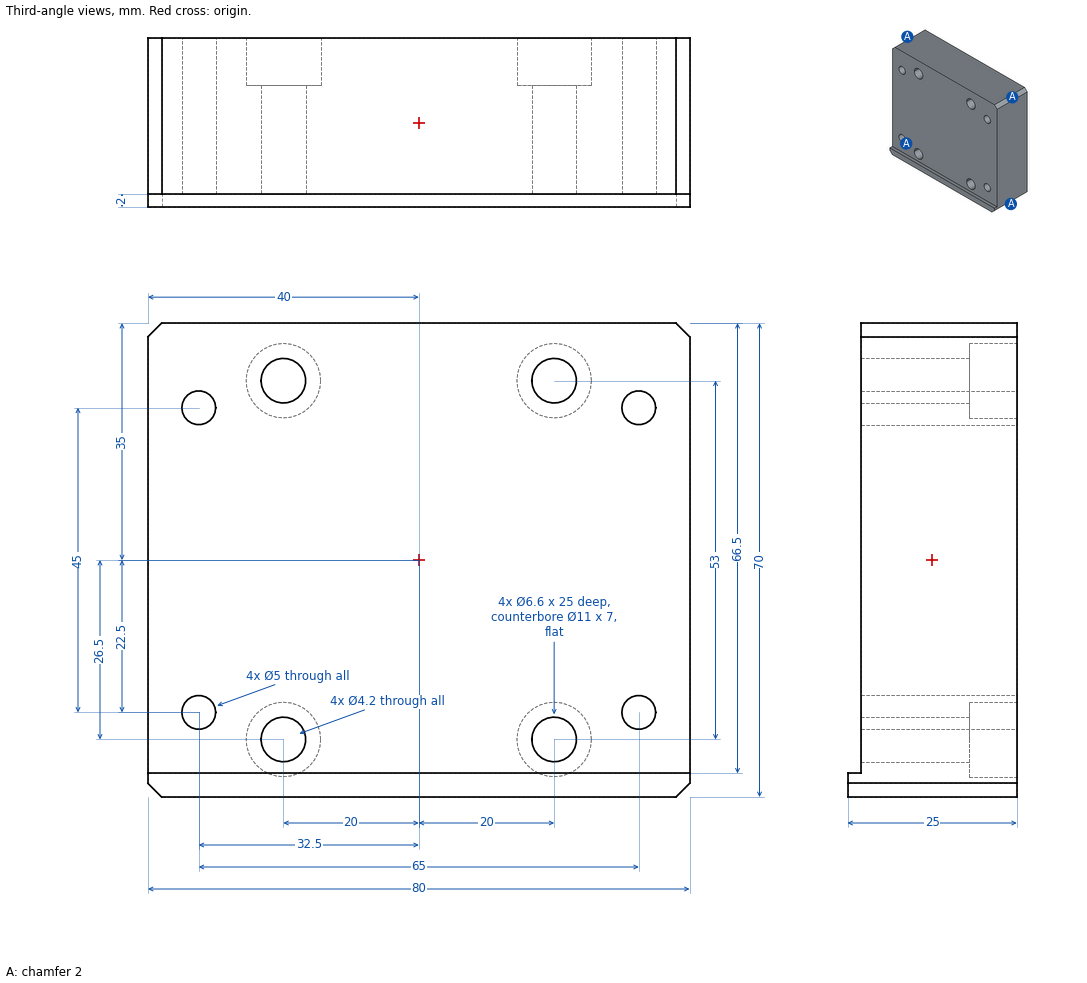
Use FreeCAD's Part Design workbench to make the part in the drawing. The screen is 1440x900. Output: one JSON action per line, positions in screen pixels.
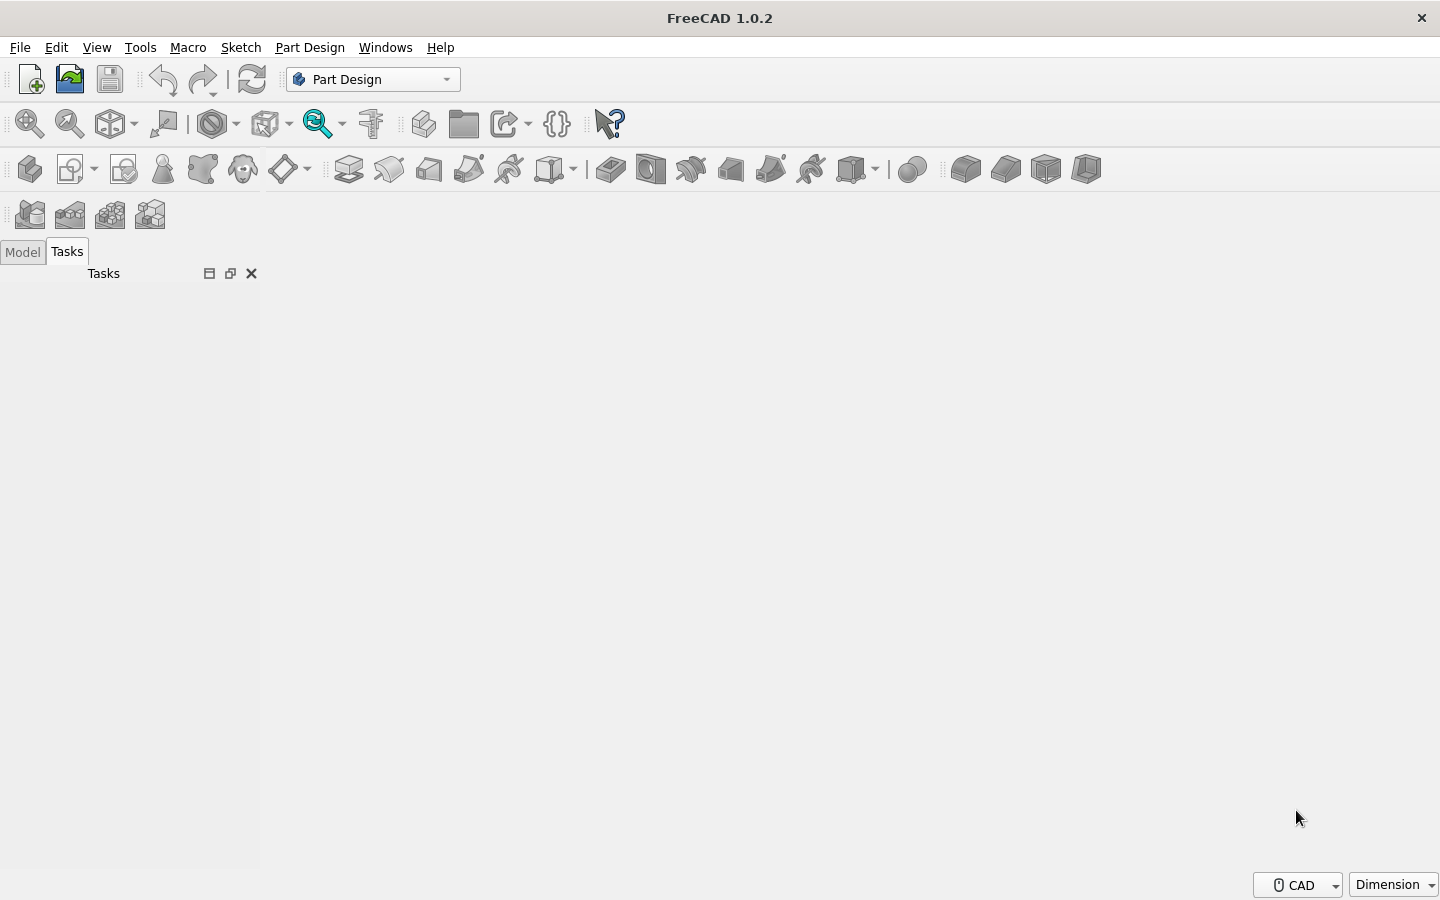
{"action": "left_click", "coordinate": [30, 80]}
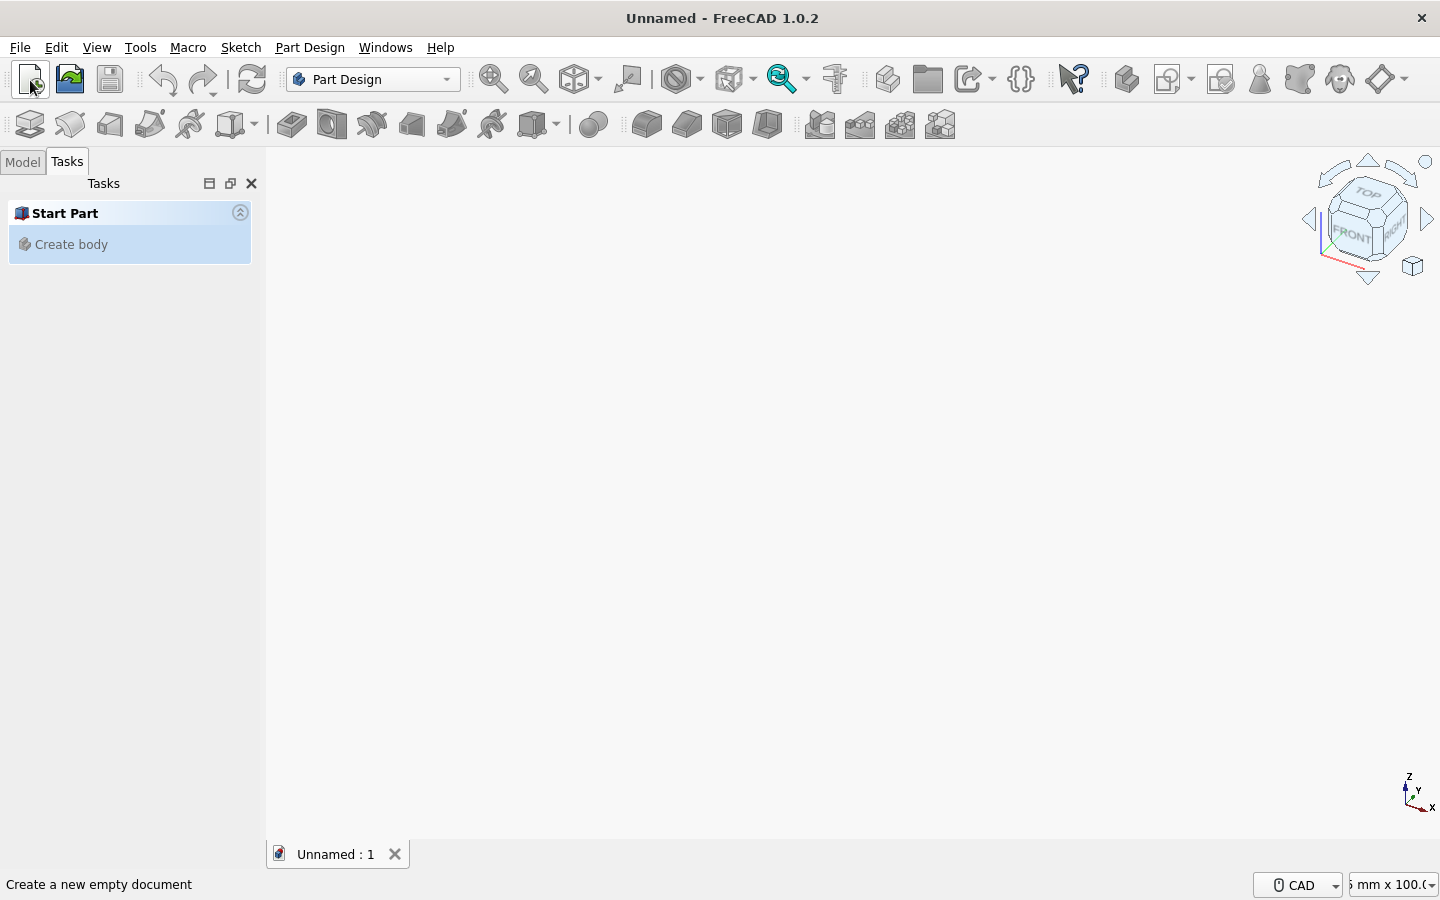
{"action": "left_click", "coordinate": [1168, 80]}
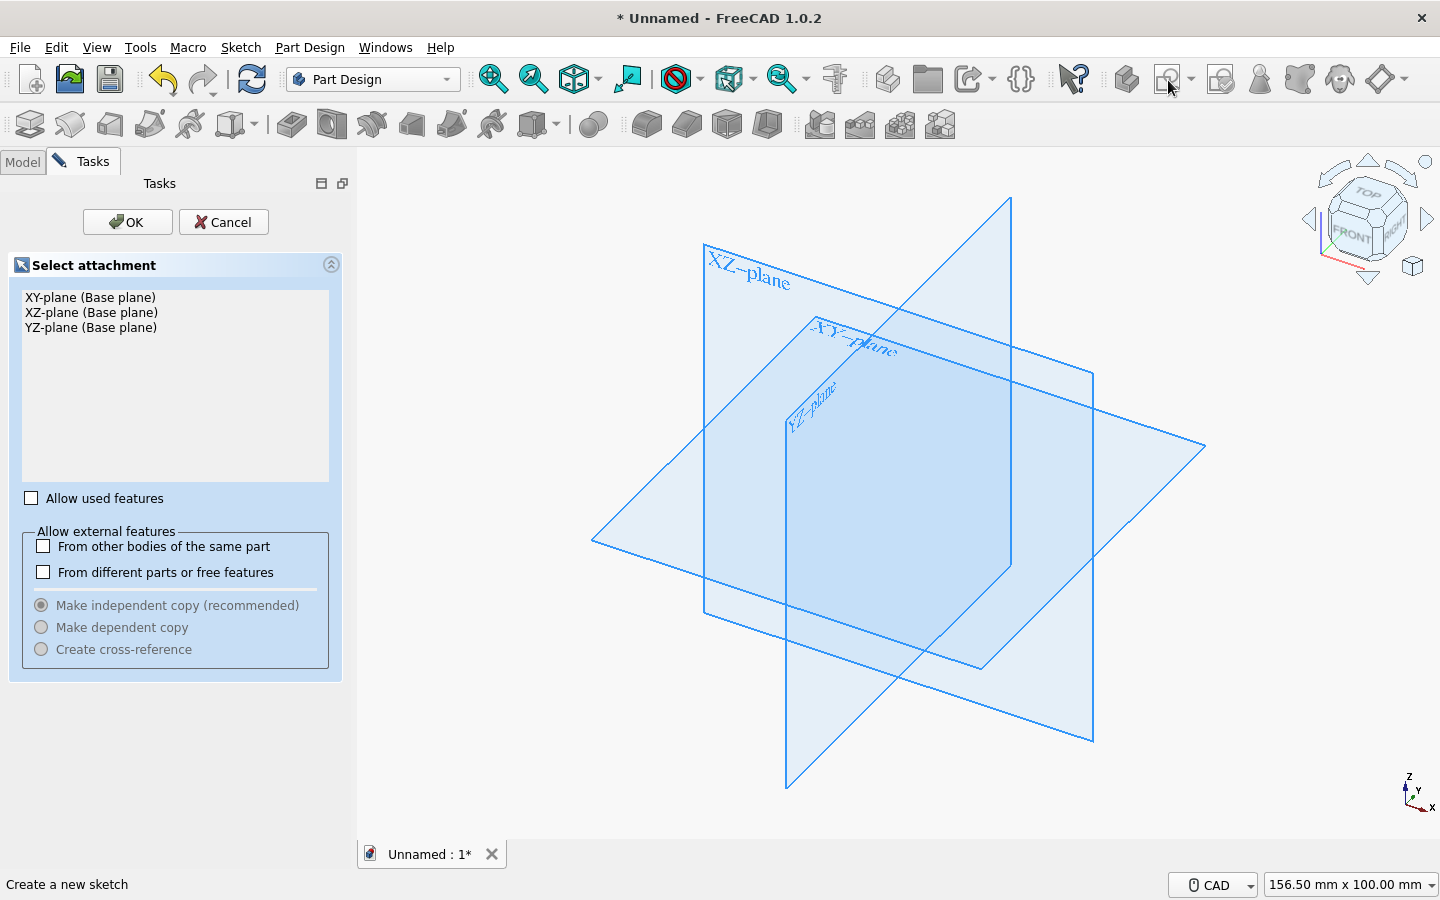
{"action": "left_click", "coordinate": [82, 312]}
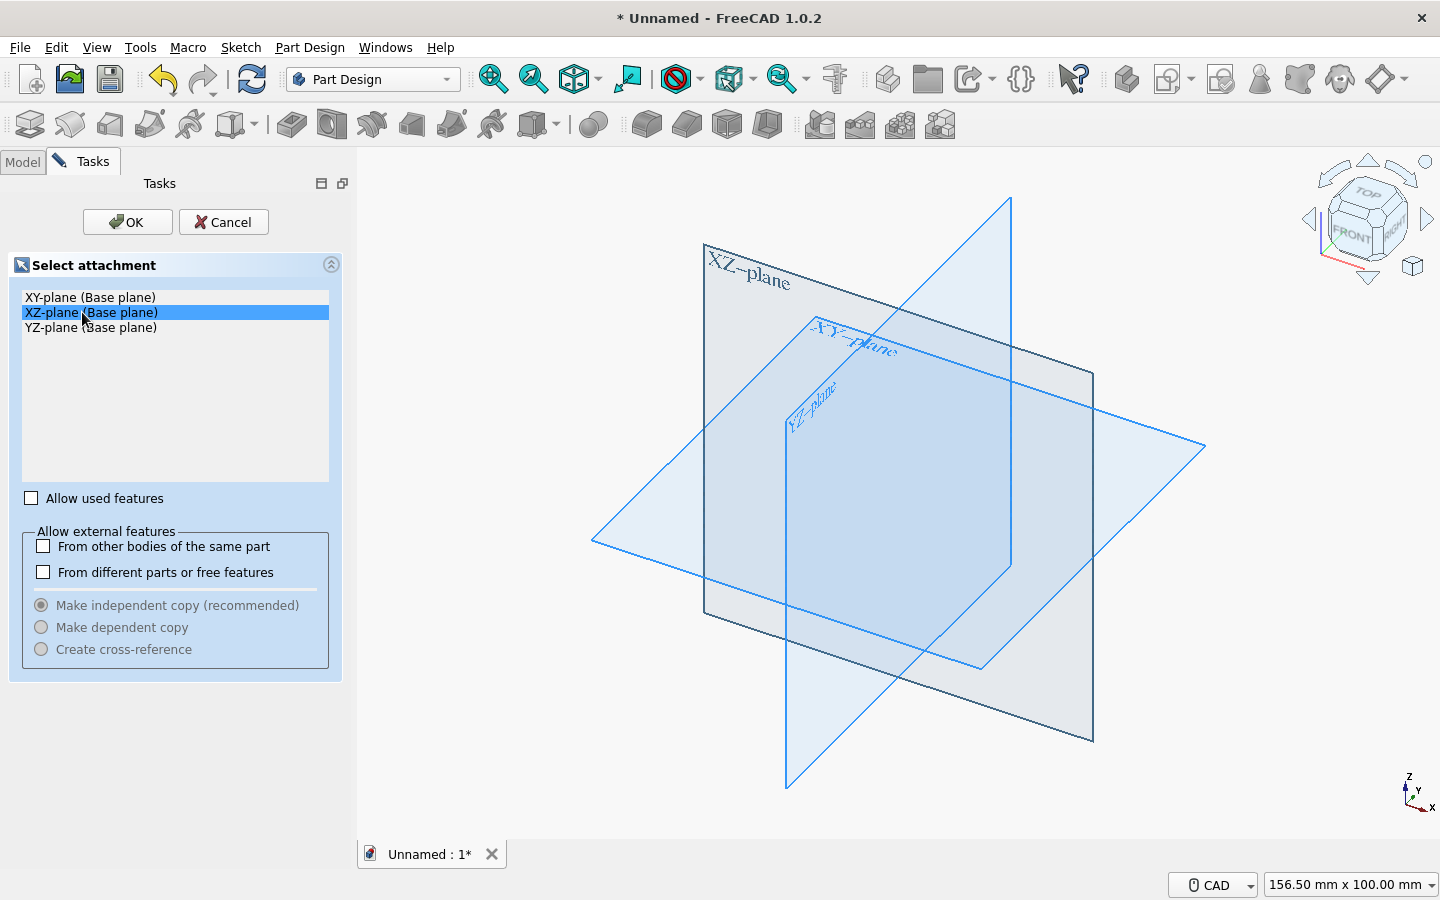
{"action": "left_click", "coordinate": [128, 222]}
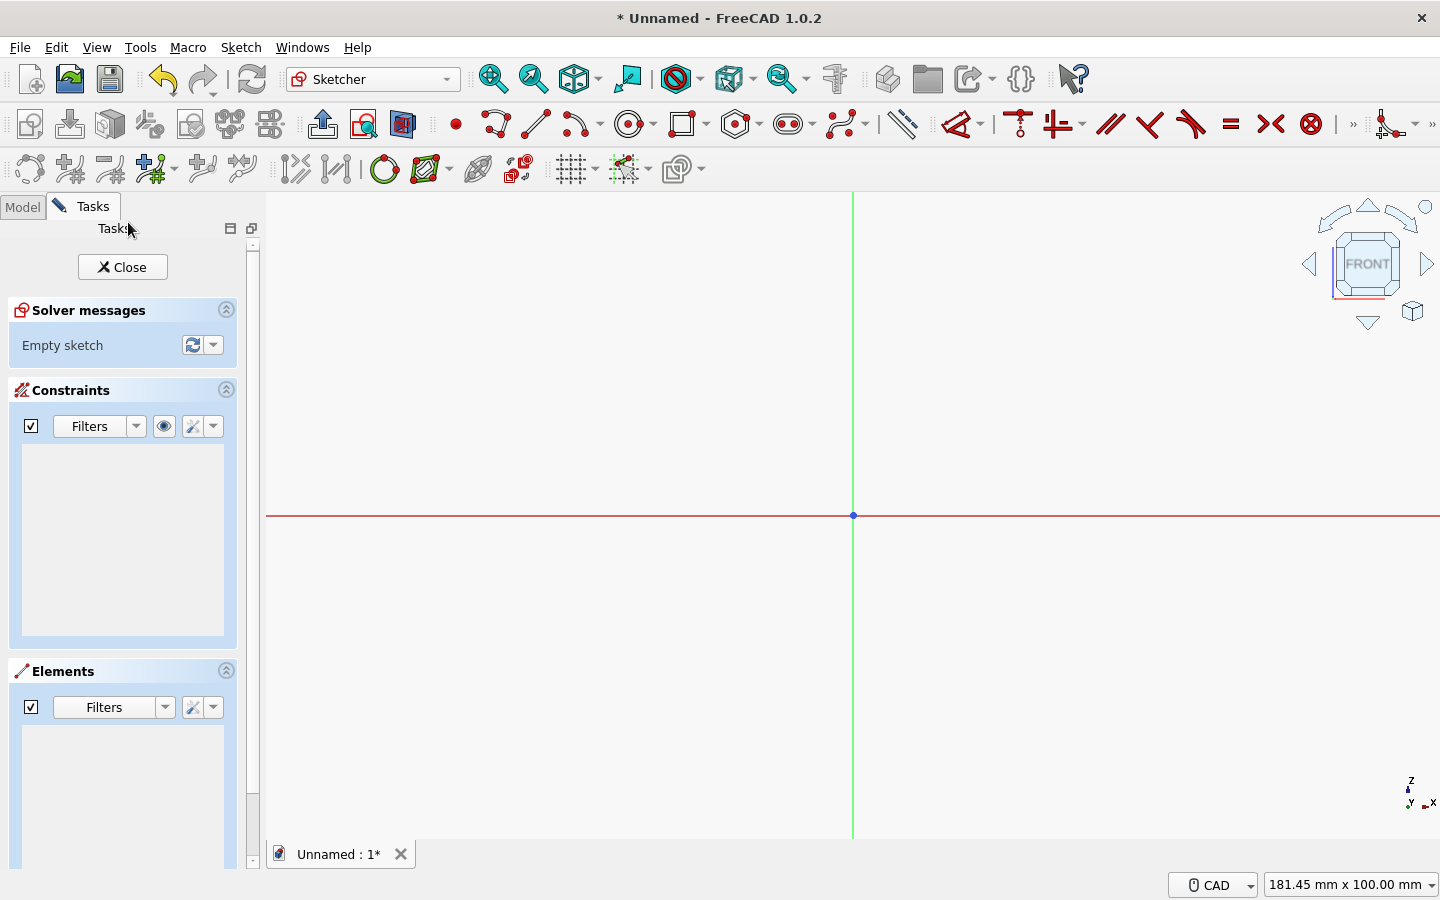
{"action": "left_click", "coordinate": [708, 124]}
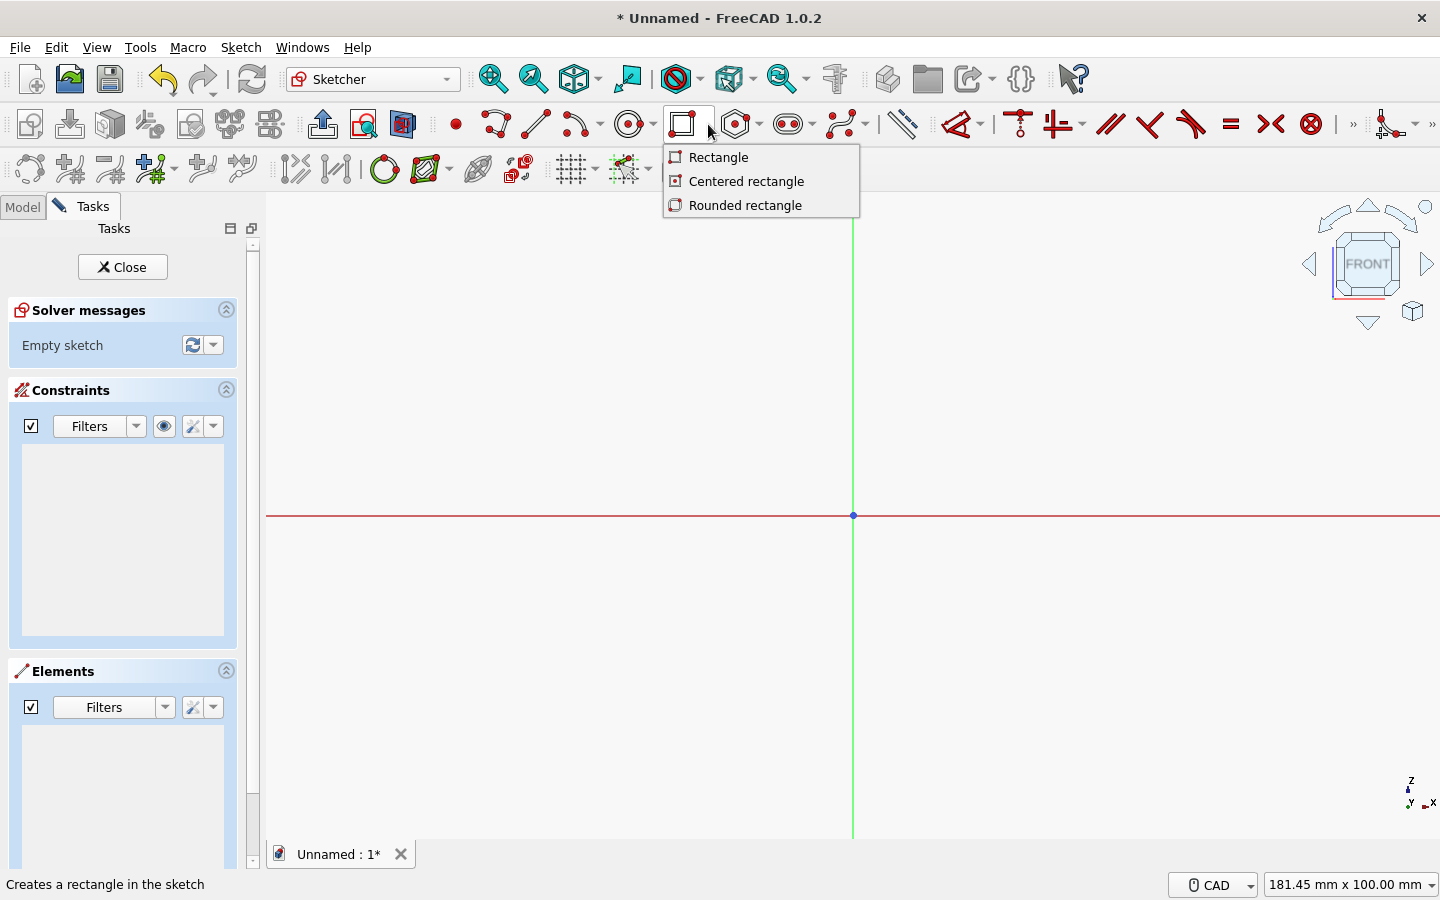
{"action": "left_click", "coordinate": [762, 181]}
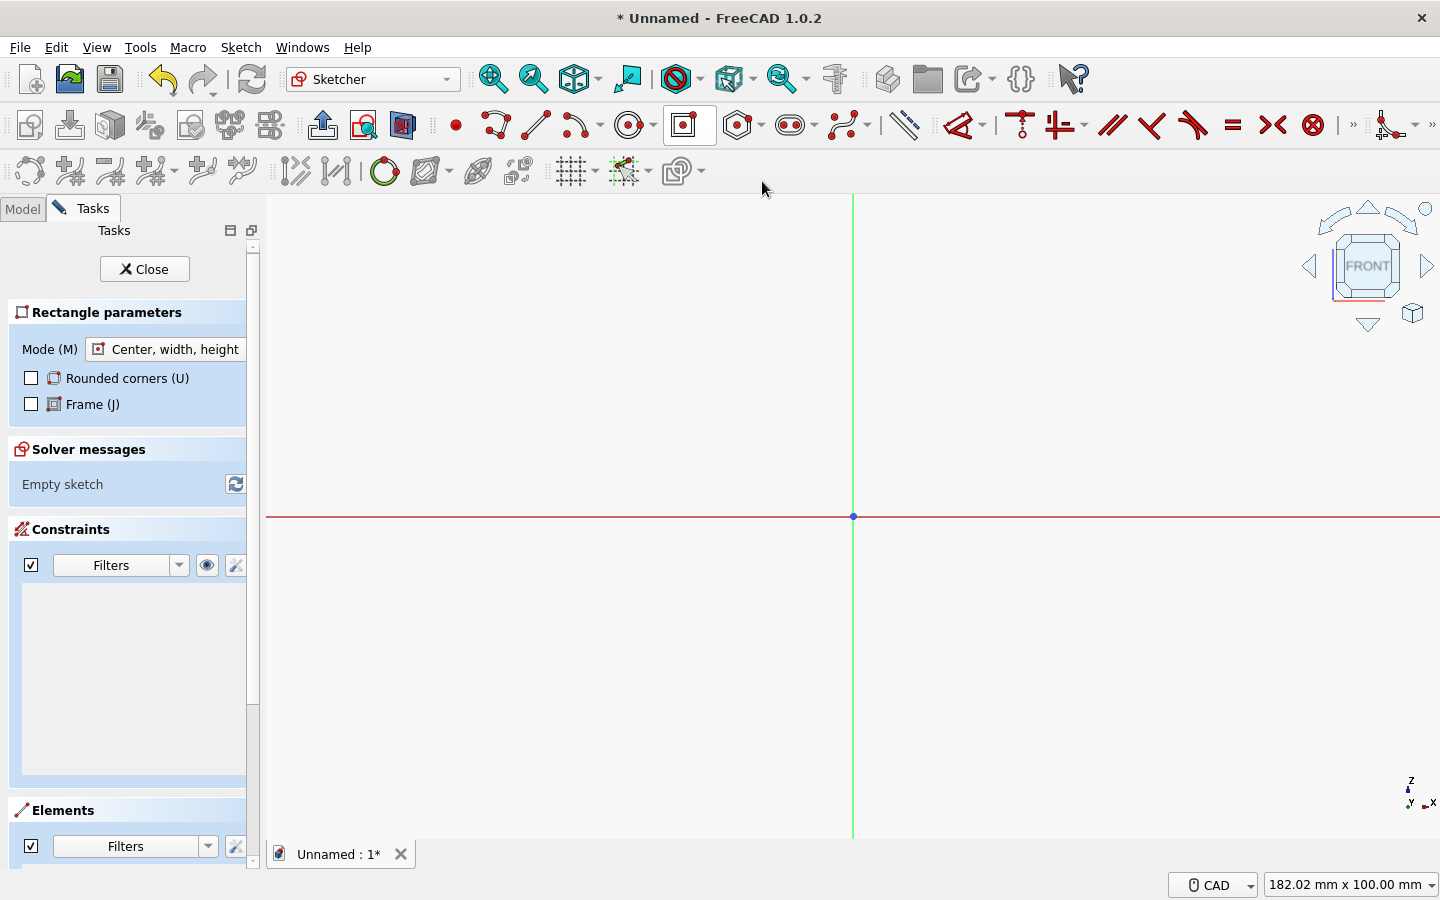
{"action": "left_click", "coordinate": [853, 516]}
{"action": "mouse_move", "coordinate": [1111, 291]}